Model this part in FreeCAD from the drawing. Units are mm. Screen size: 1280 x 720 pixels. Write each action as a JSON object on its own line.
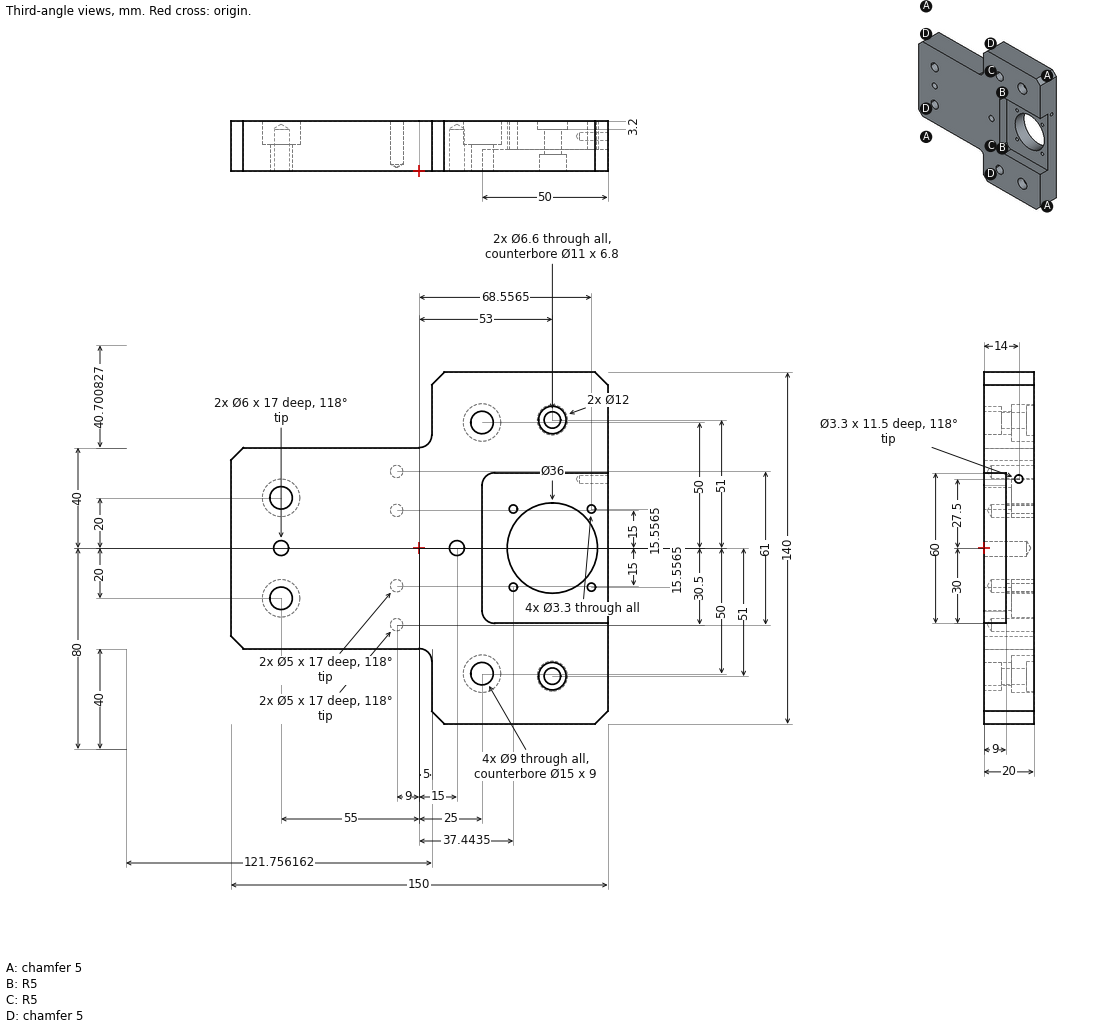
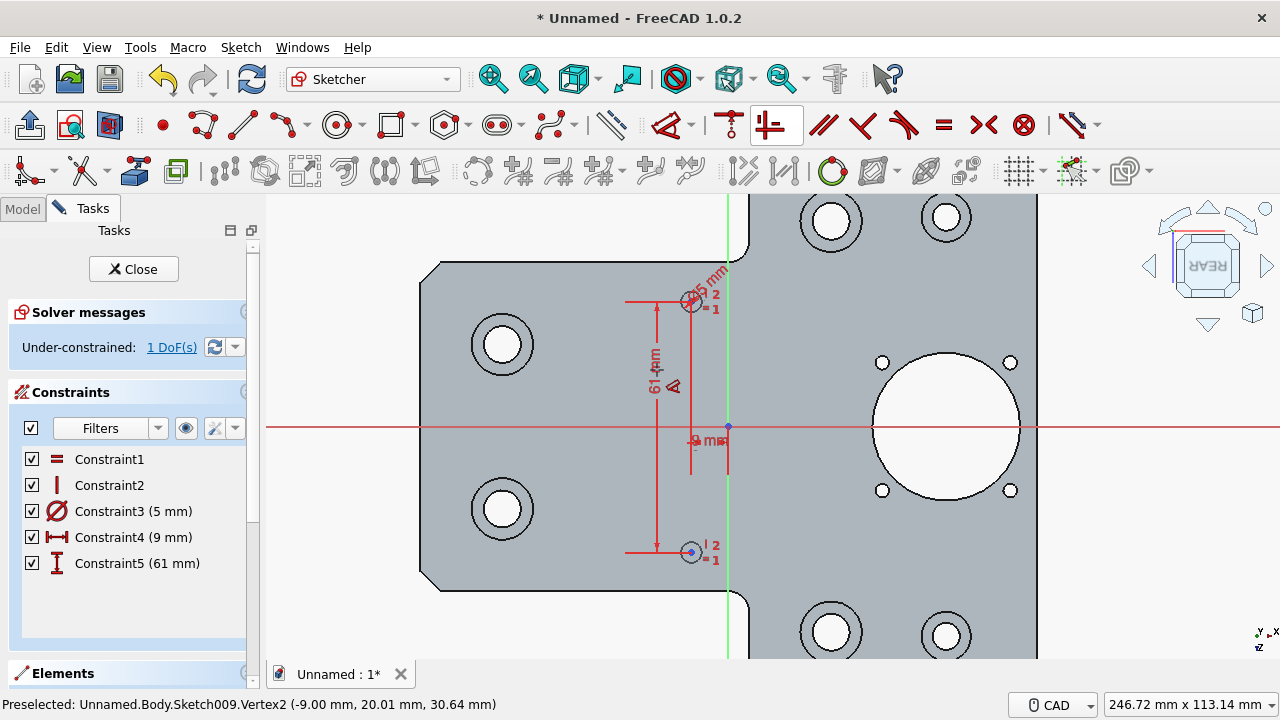
{"action": "left_click", "coordinate": [691, 302]}
{"action": "left_click", "coordinate": [762, 364]}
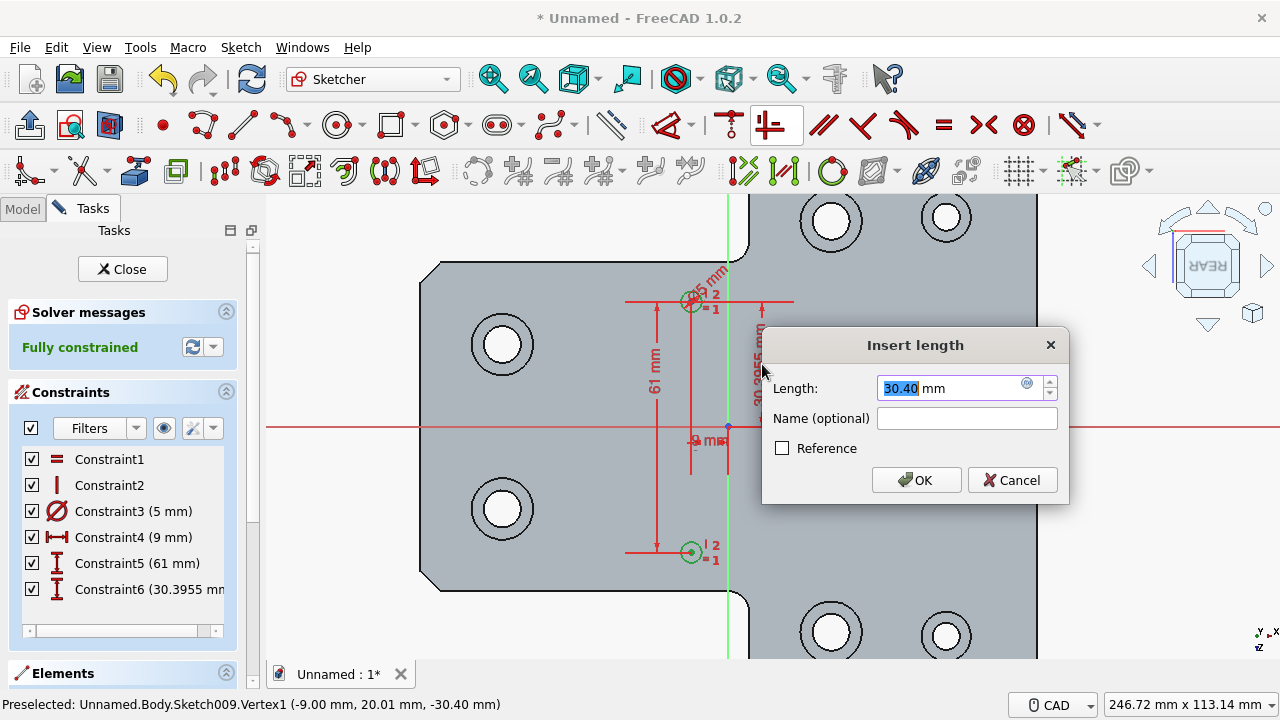
{"action": "type", "text": "30.5"}
{"action": "key", "text": "Return"}
{"action": "key", "text": "Escape"}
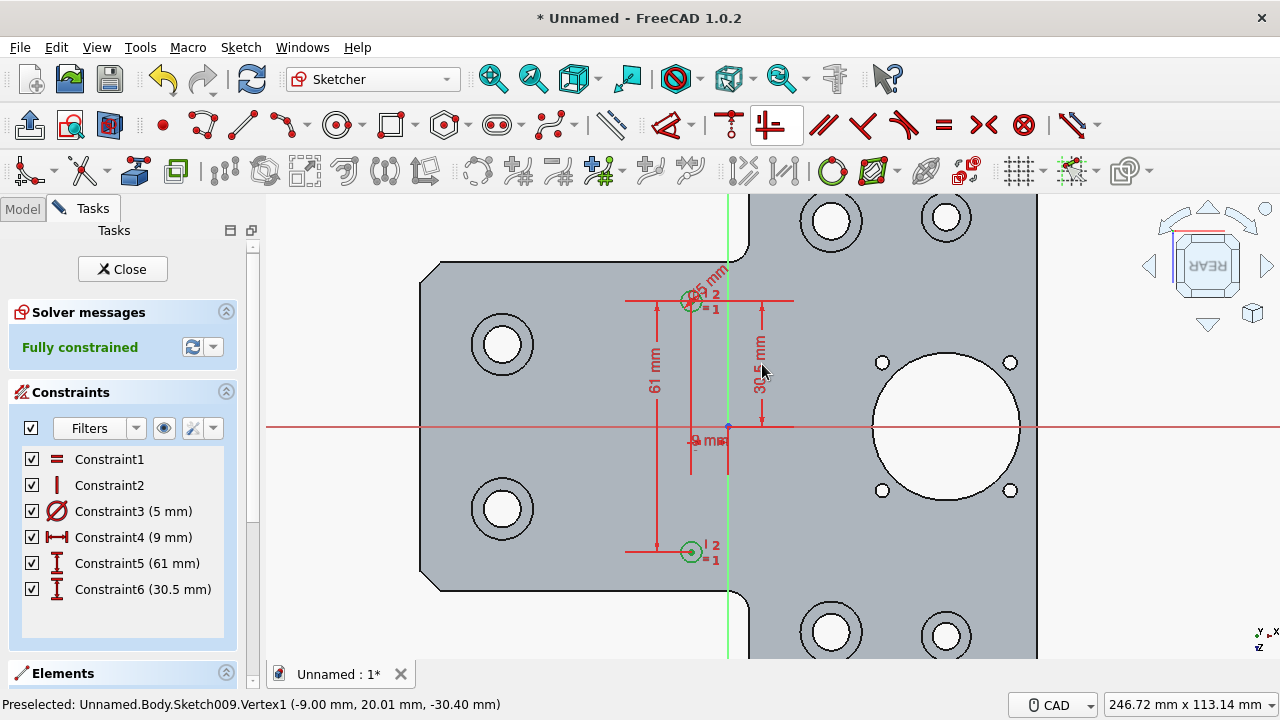
{"action": "left_click", "coordinate": [123, 269]}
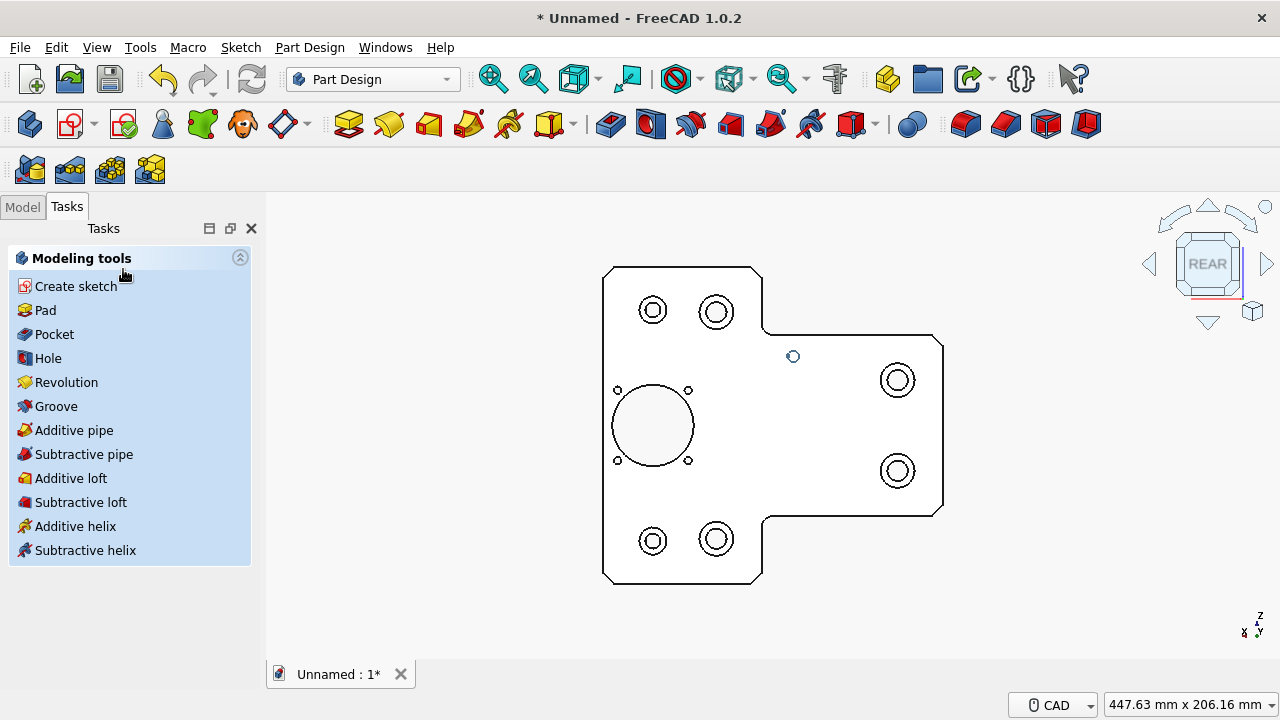
{"action": "left_click", "coordinate": [652, 124]}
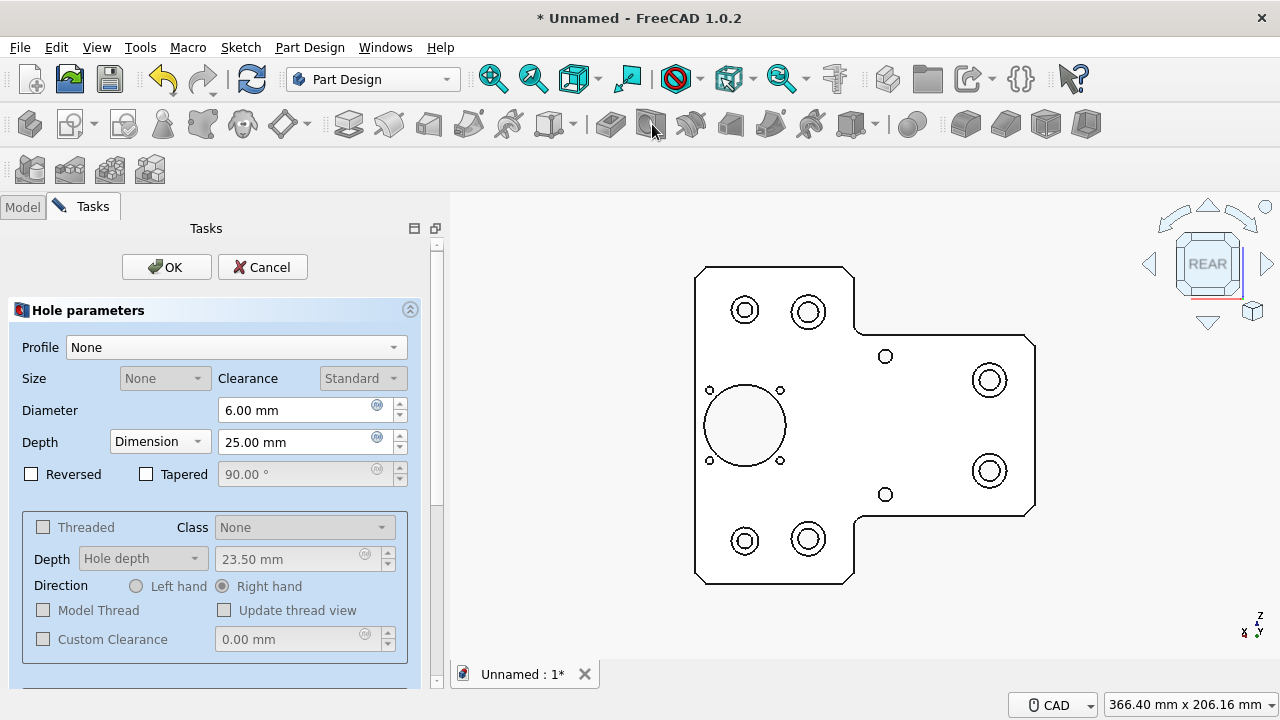
{"action": "triple_click", "coordinate": [305, 410]}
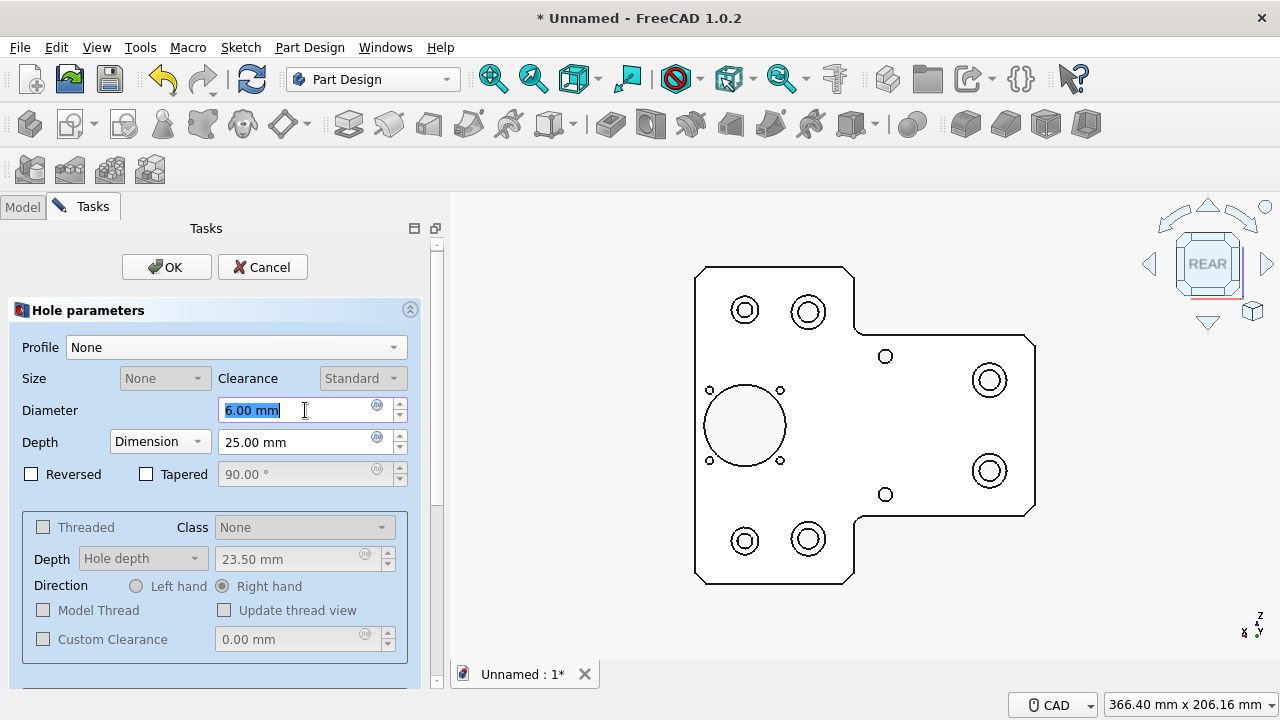
{"action": "type", "text": "5"}
{"action": "key", "text": "Tab"}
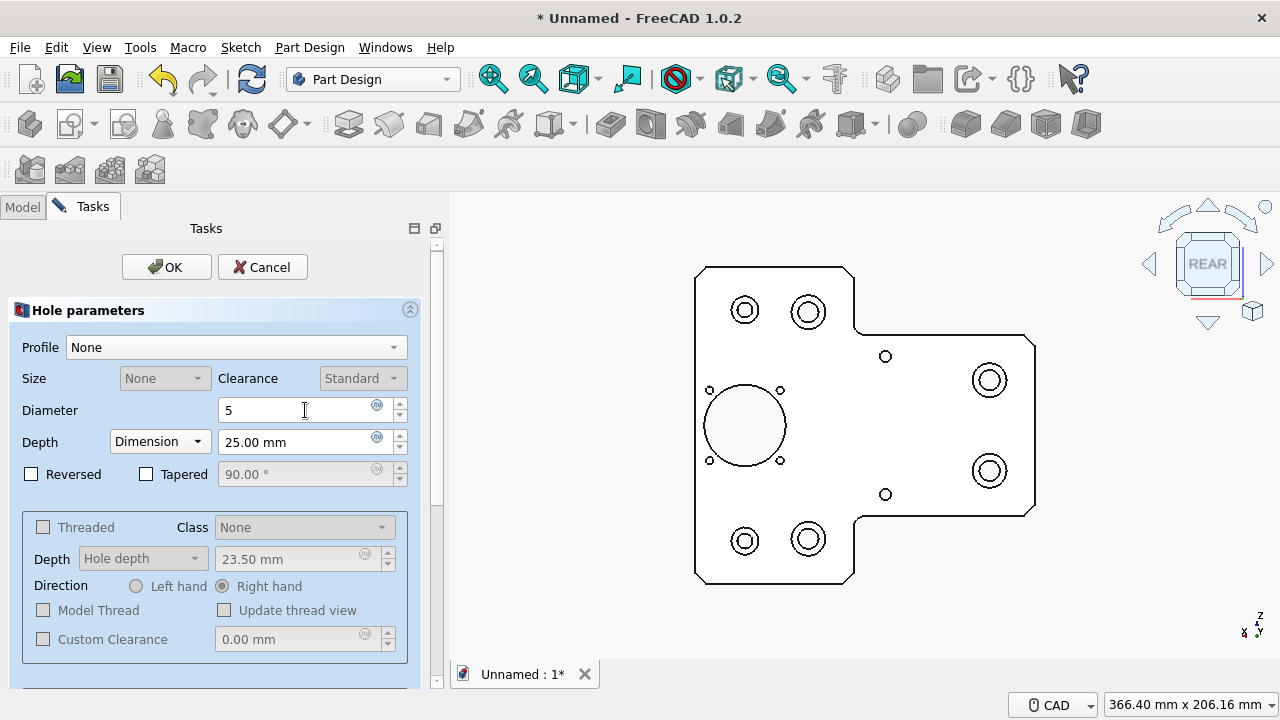
{"action": "triple_click", "coordinate": [305, 442]}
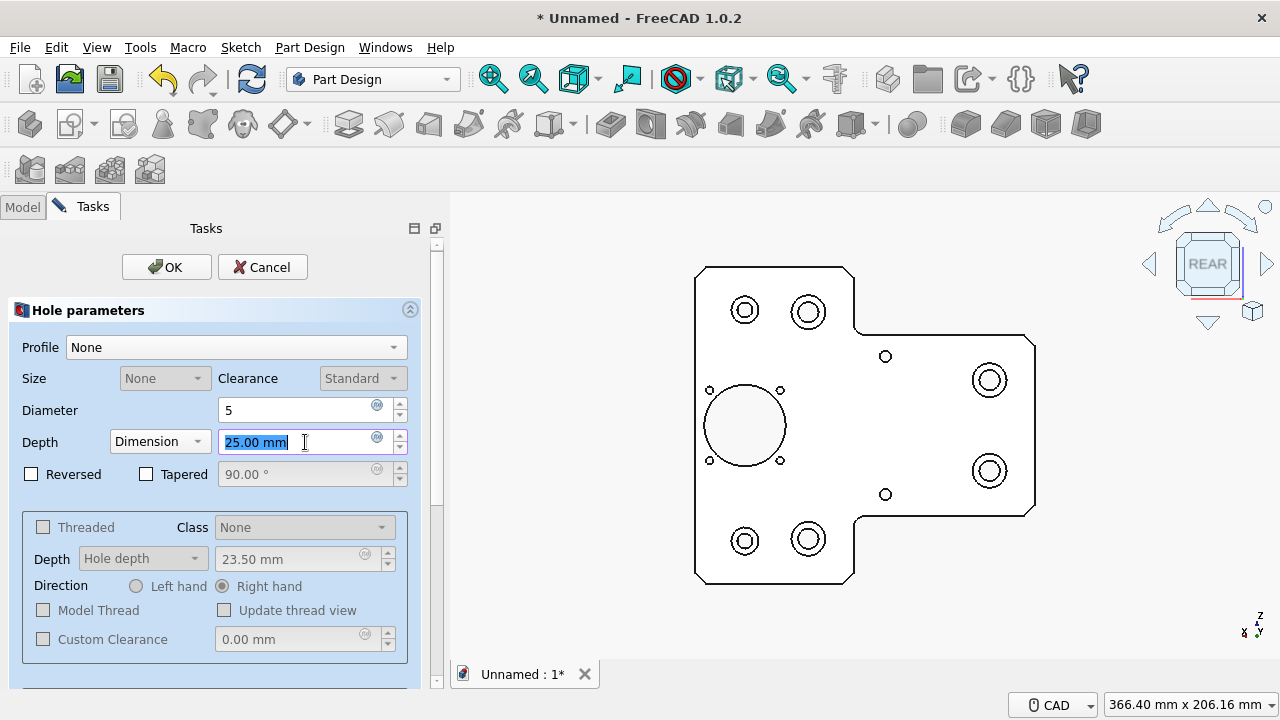
{"action": "type", "text": "17"}
{"action": "key", "text": "Tab"}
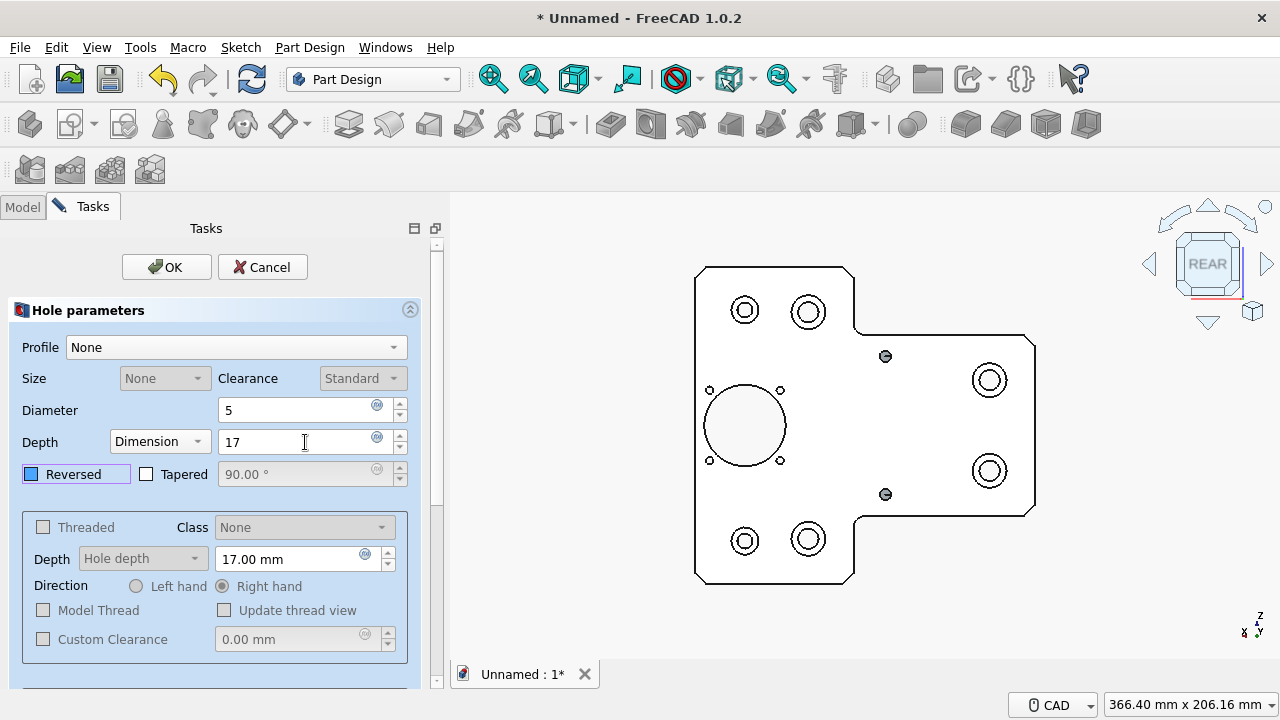
{"action": "left_click", "coordinate": [167, 267]}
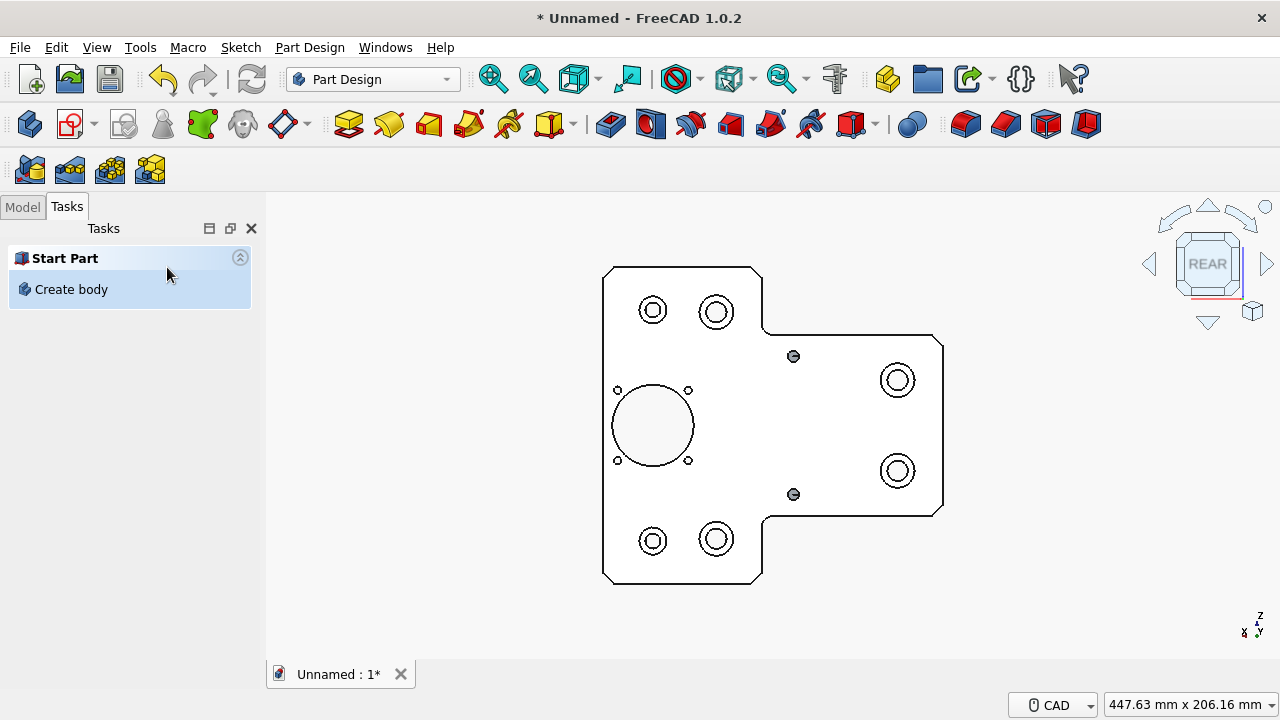
{"action": "left_click", "coordinate": [822, 424]}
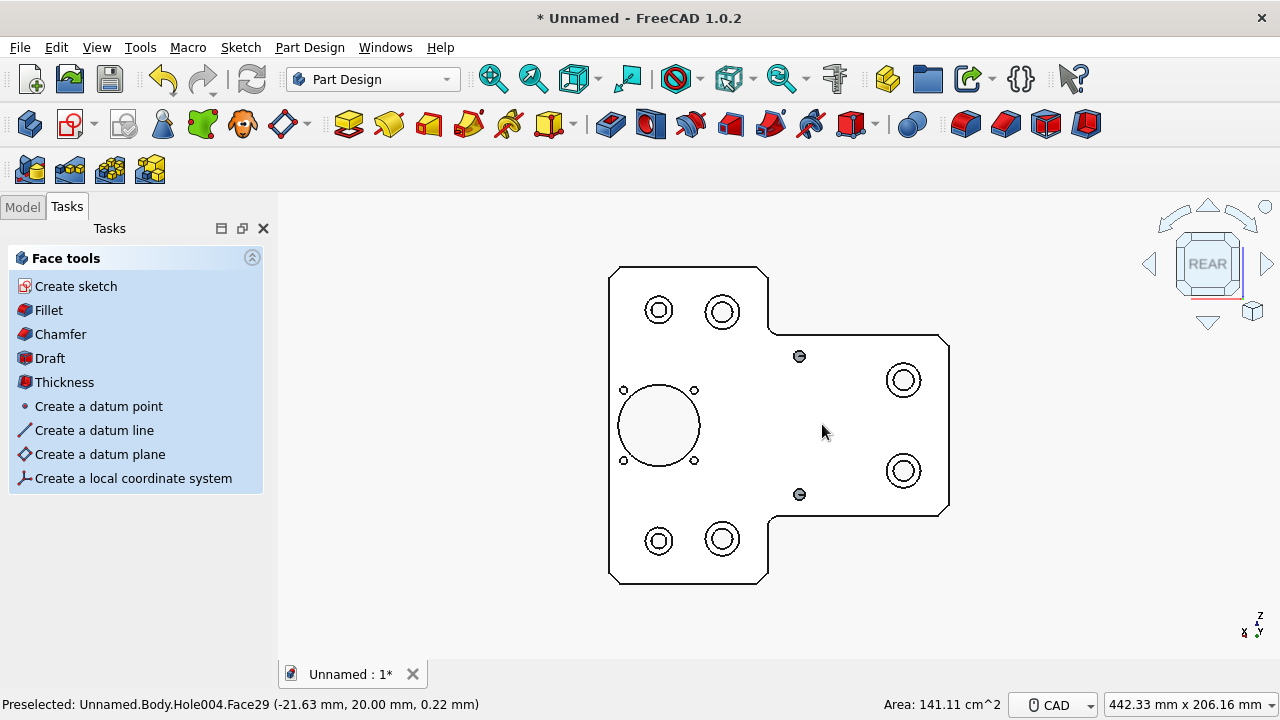
{"action": "left_click", "coordinate": [70, 124]}